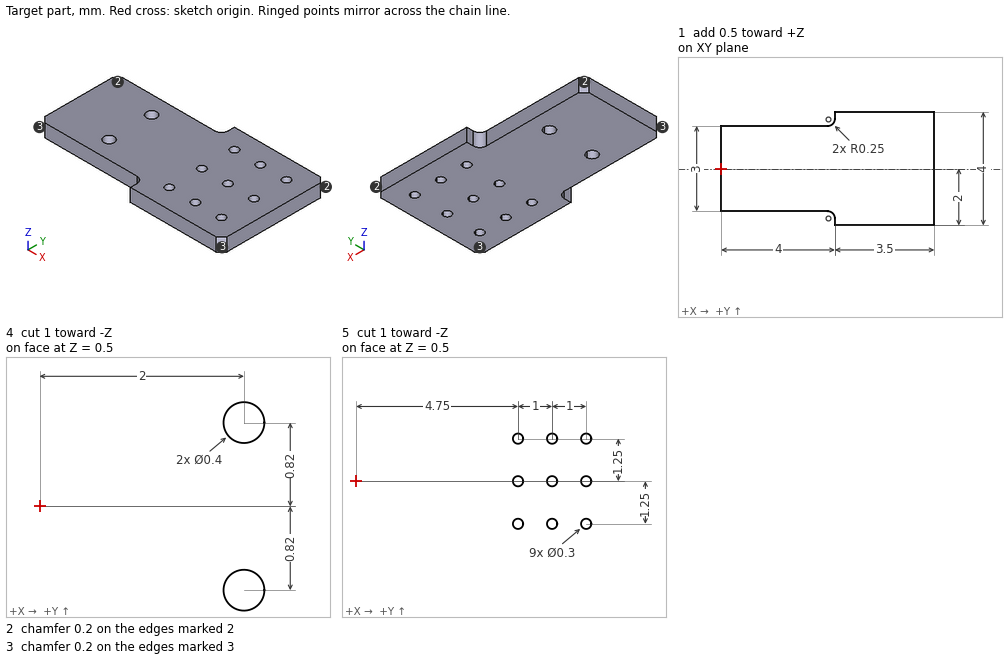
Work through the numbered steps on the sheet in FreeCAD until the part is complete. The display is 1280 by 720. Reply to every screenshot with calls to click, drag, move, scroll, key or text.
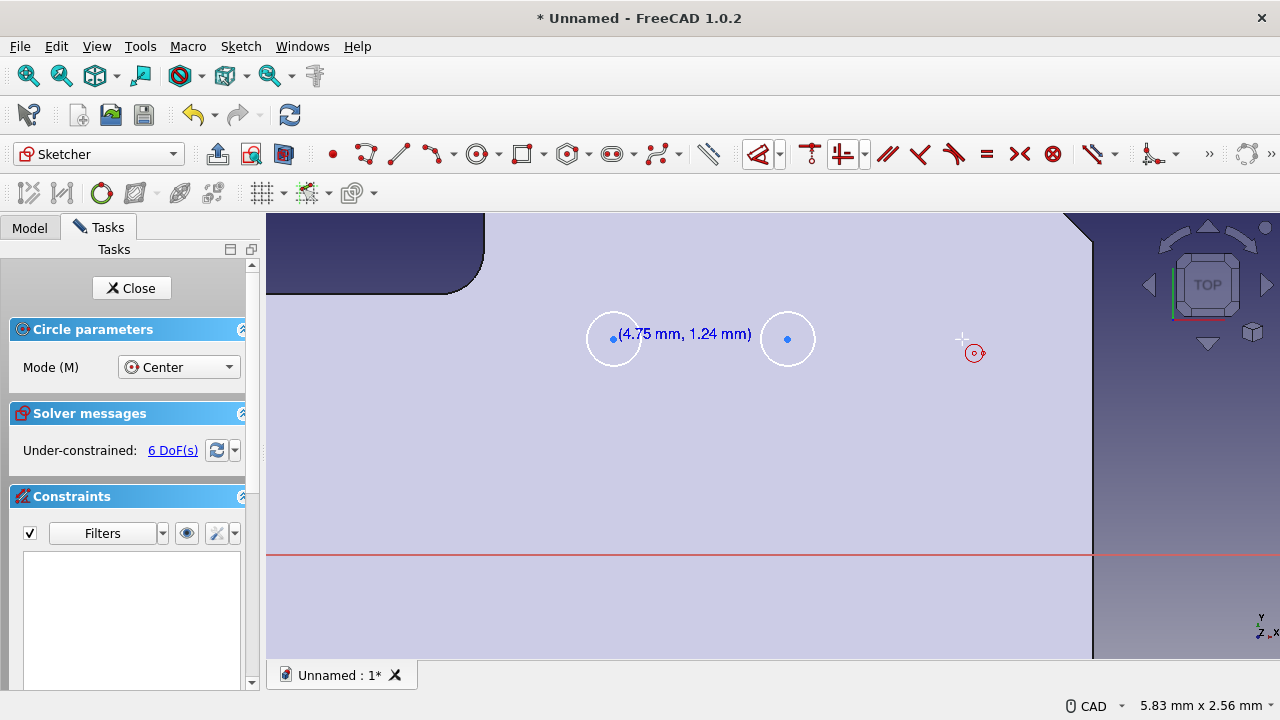
click(962, 338)
click(981, 319)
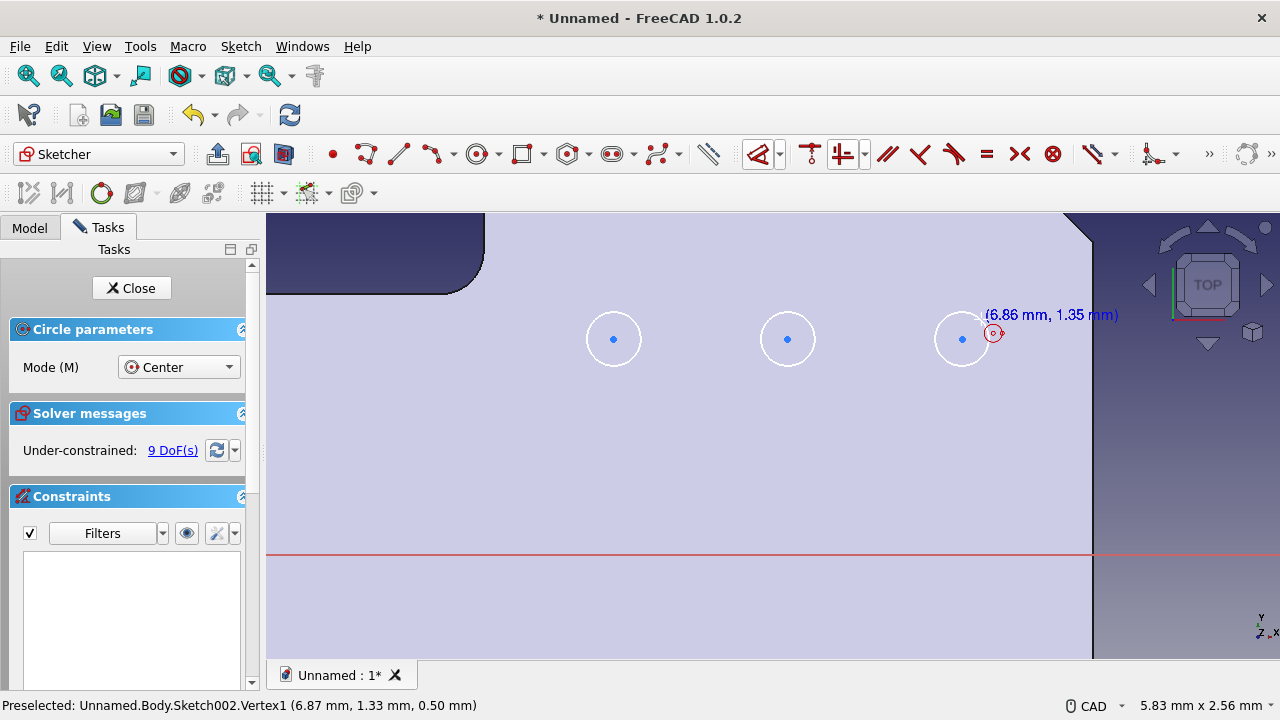
click(962, 555)
click(981, 537)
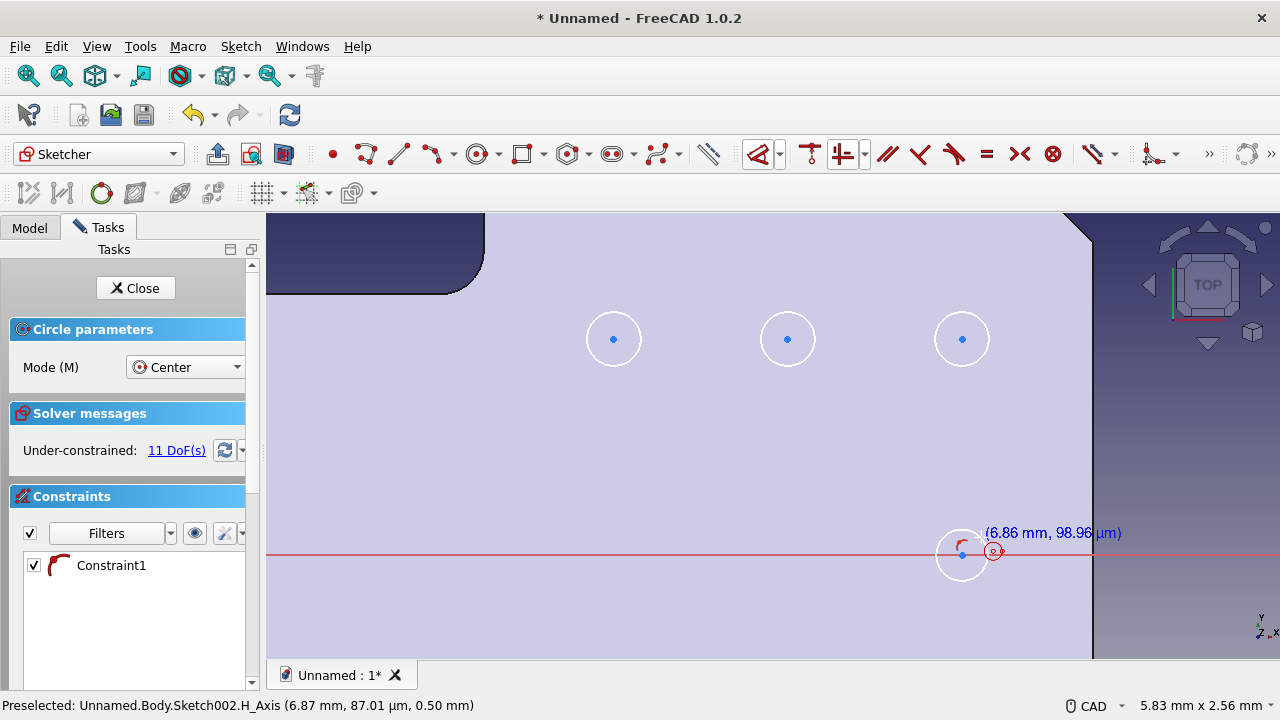
scroll(963, 339, down, 4)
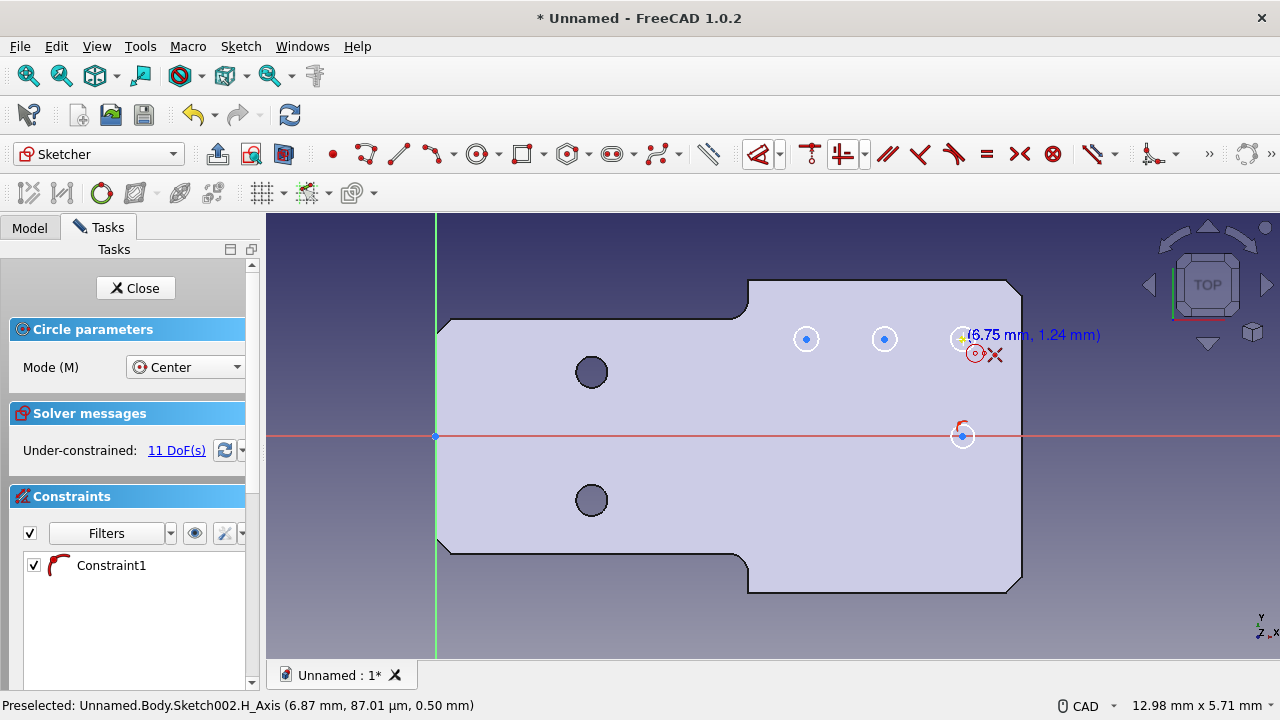
scroll(963, 534, up, 4)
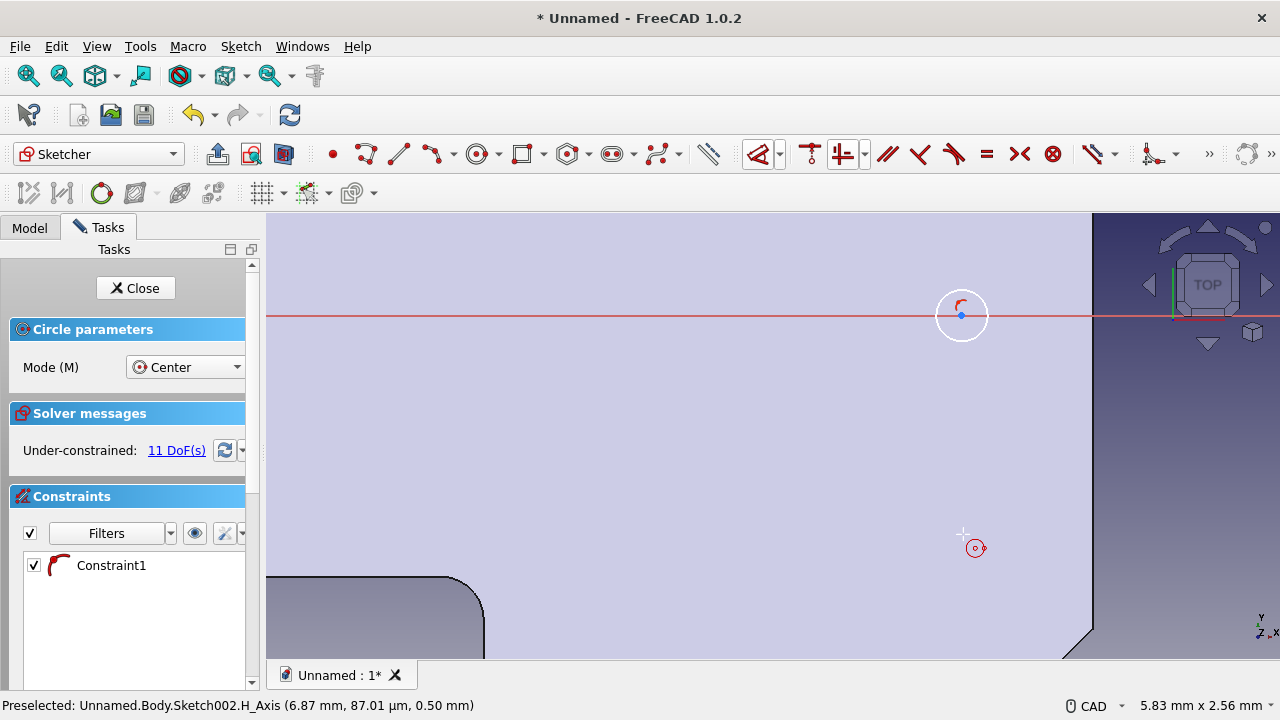
click(962, 533)
click(981, 515)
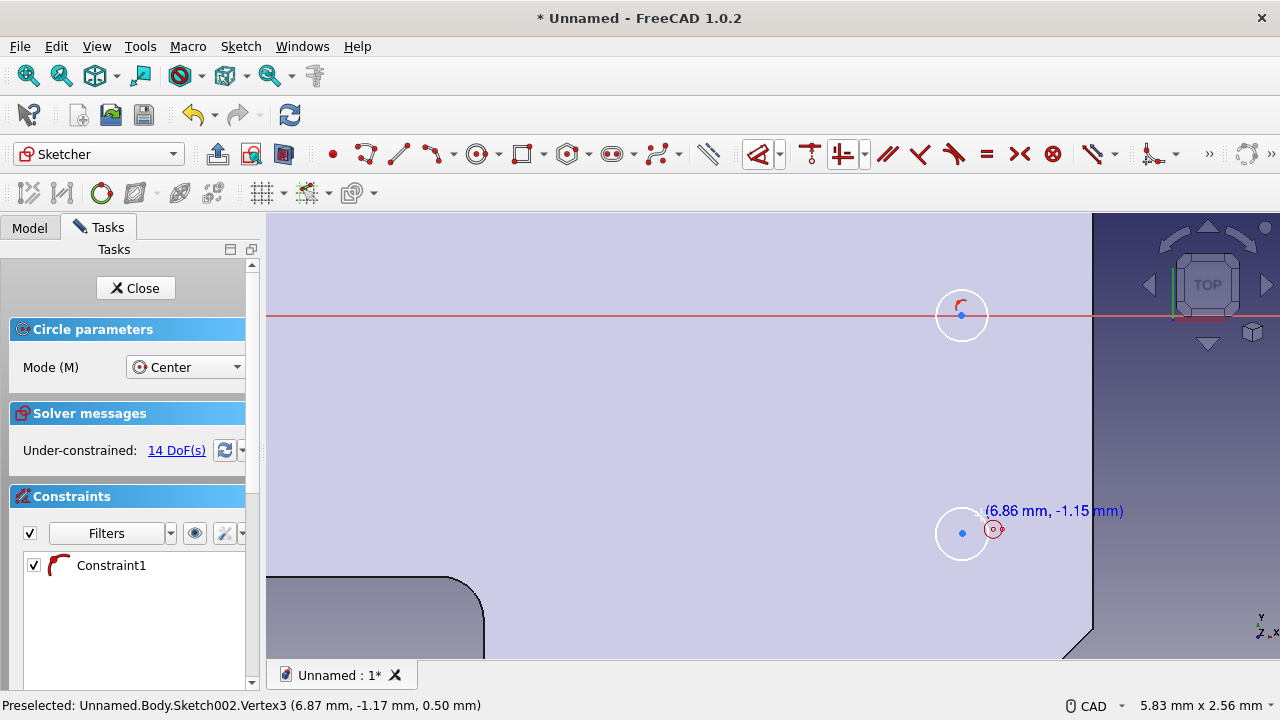
click(788, 533)
click(807, 515)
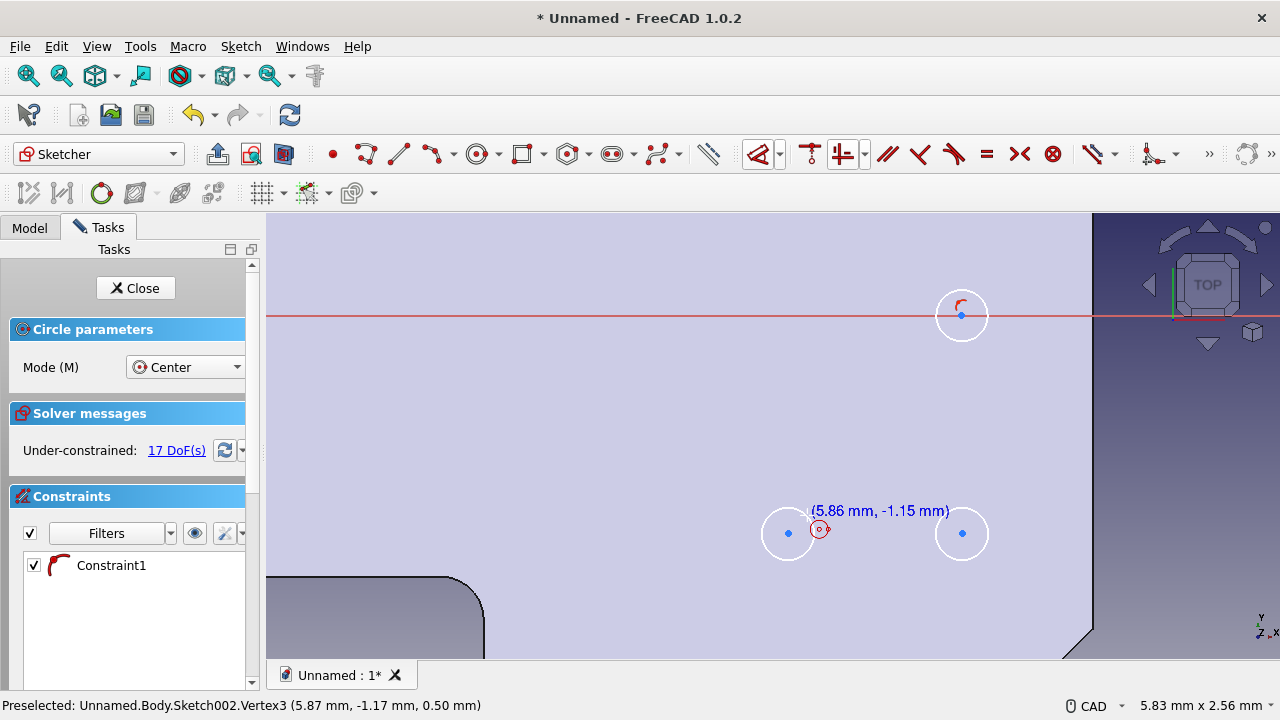
click(614, 533)
click(633, 515)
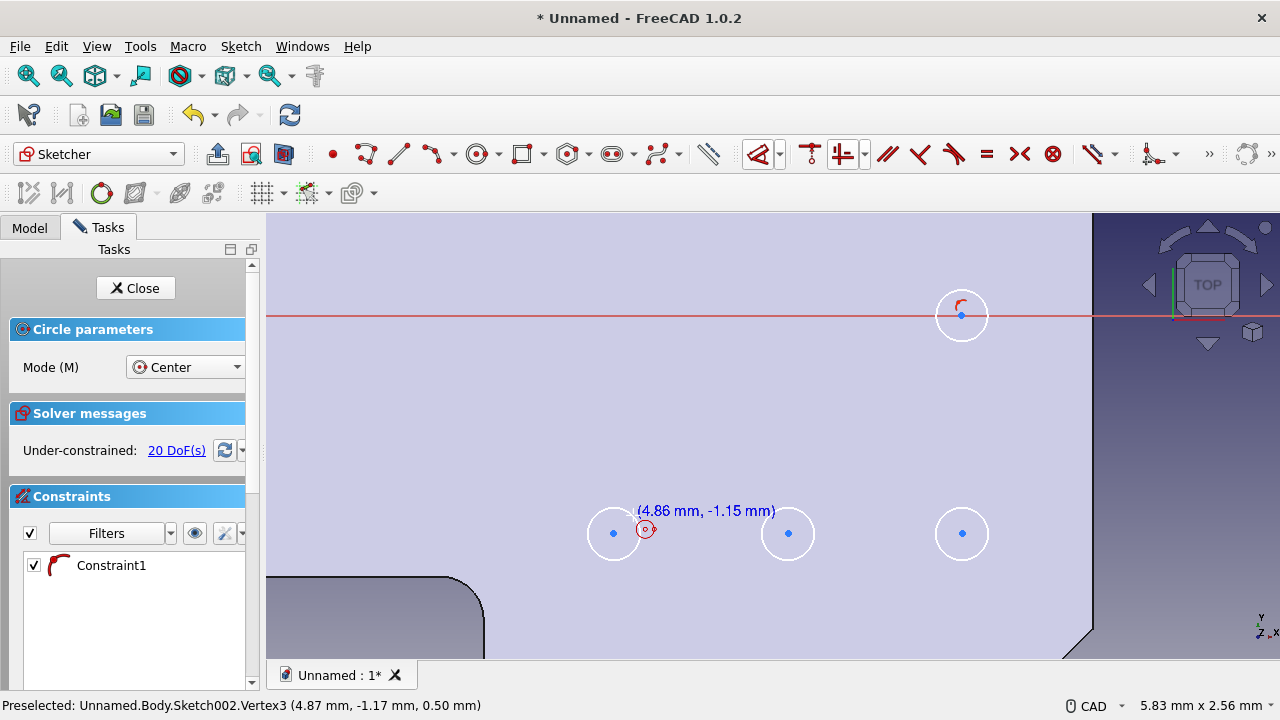
click(614, 316)
click(633, 297)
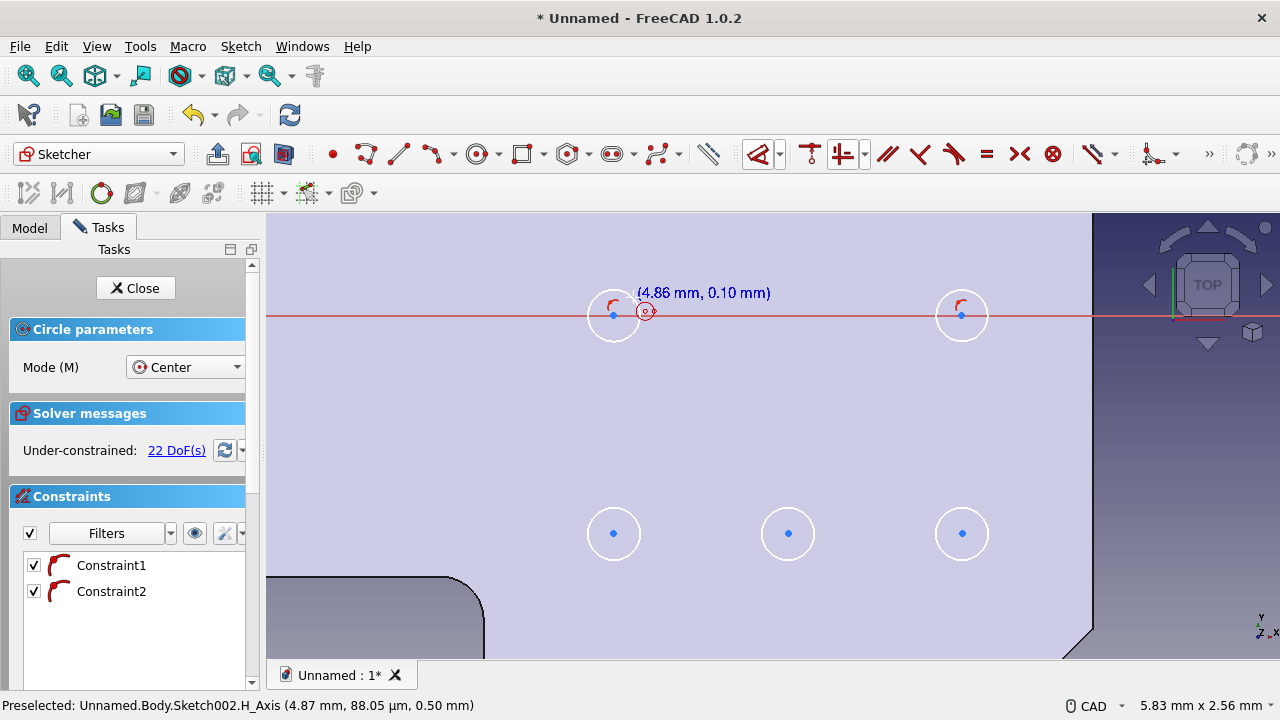
click(788, 316)
click(807, 297)
key(Escape)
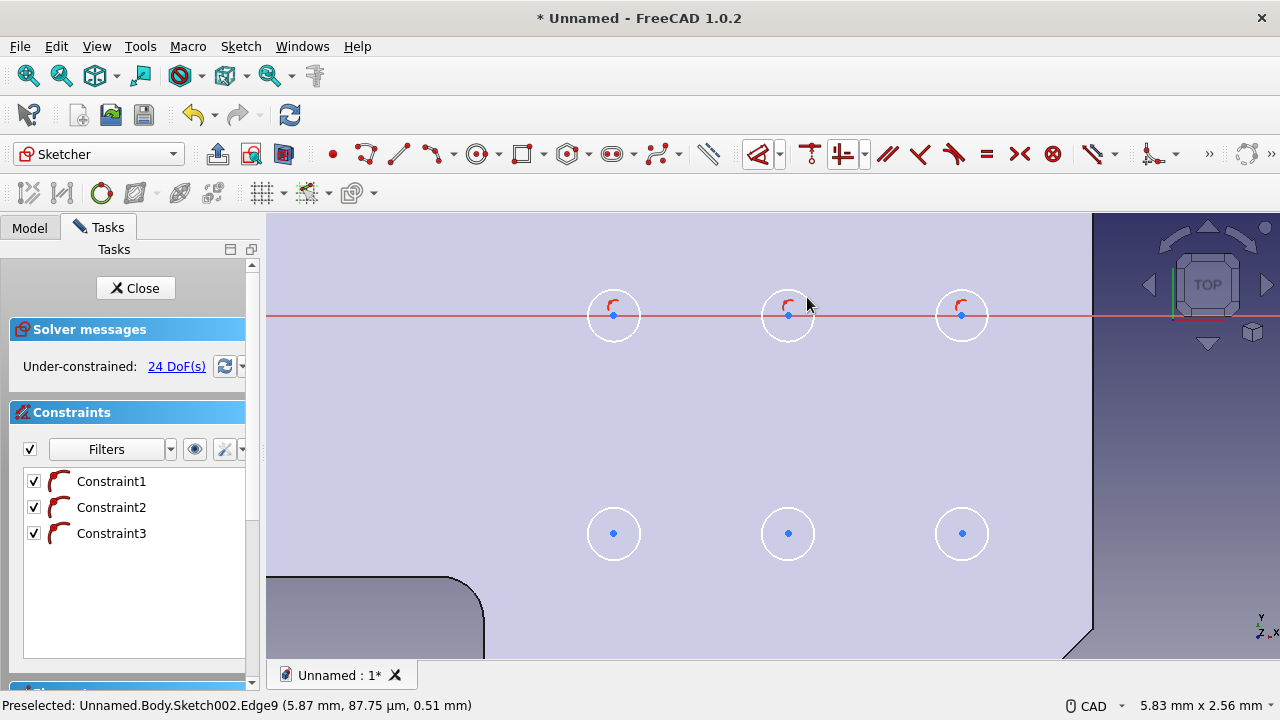
scroll(963, 534, down, 4)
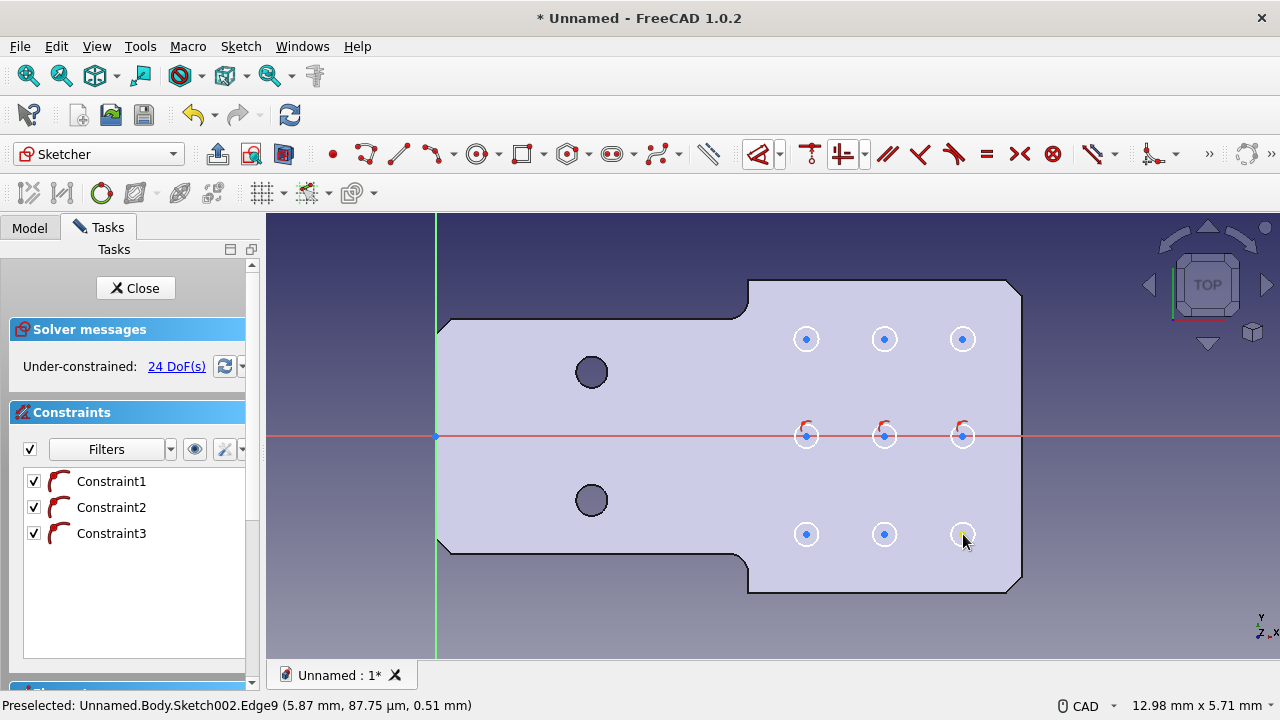
click(815, 331)